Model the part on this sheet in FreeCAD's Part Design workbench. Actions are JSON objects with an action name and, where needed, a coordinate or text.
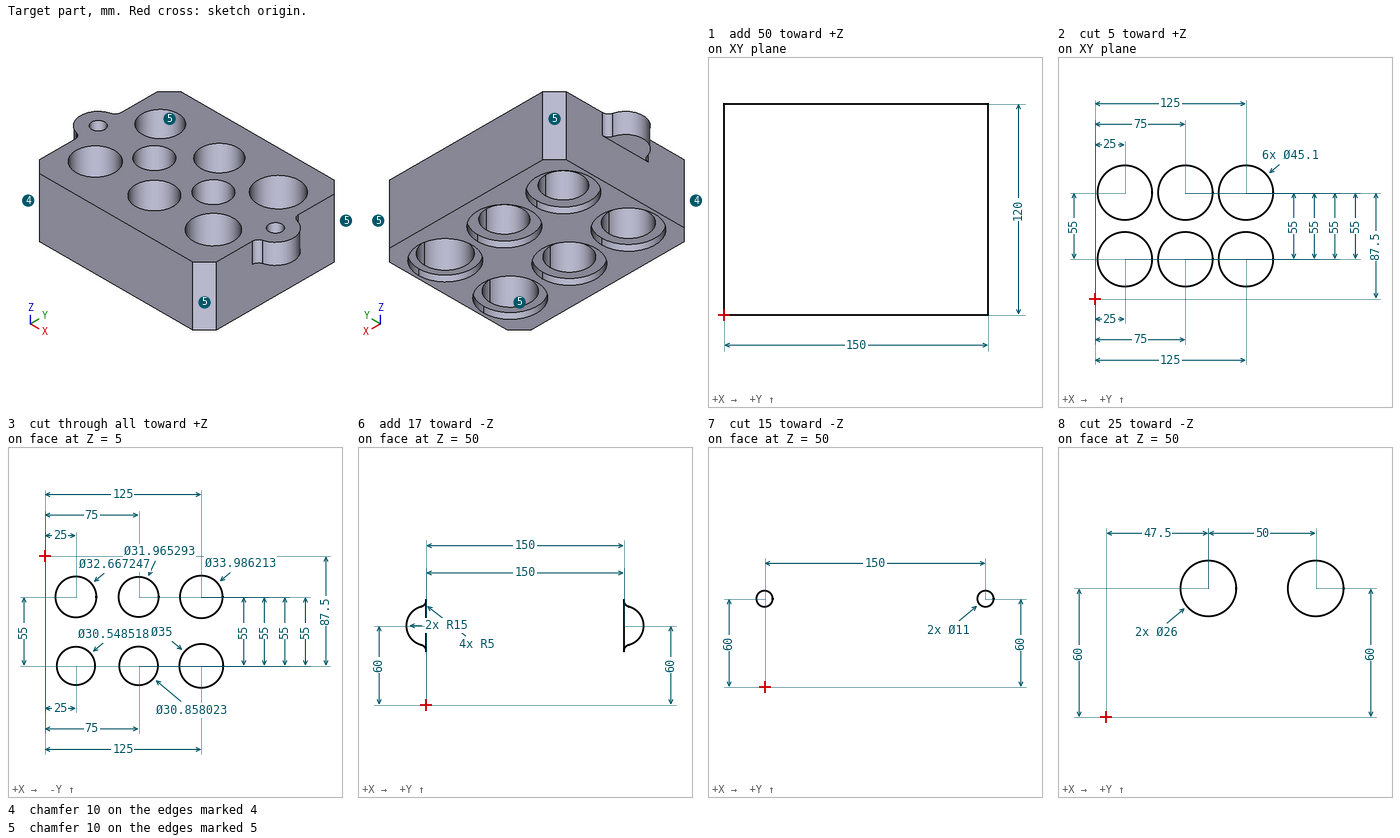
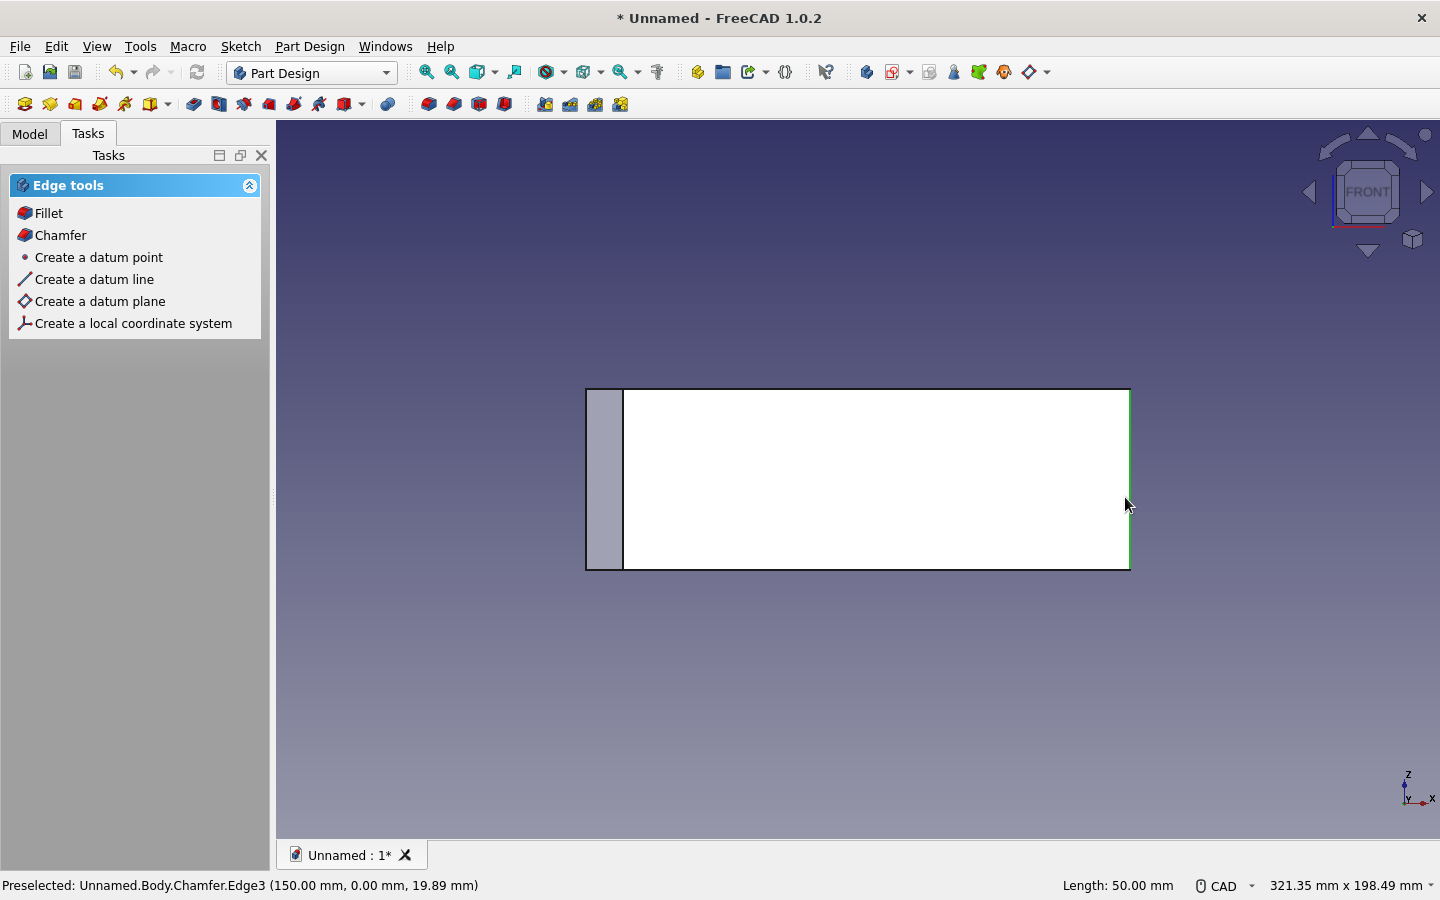
{"action": "key", "text": "3"}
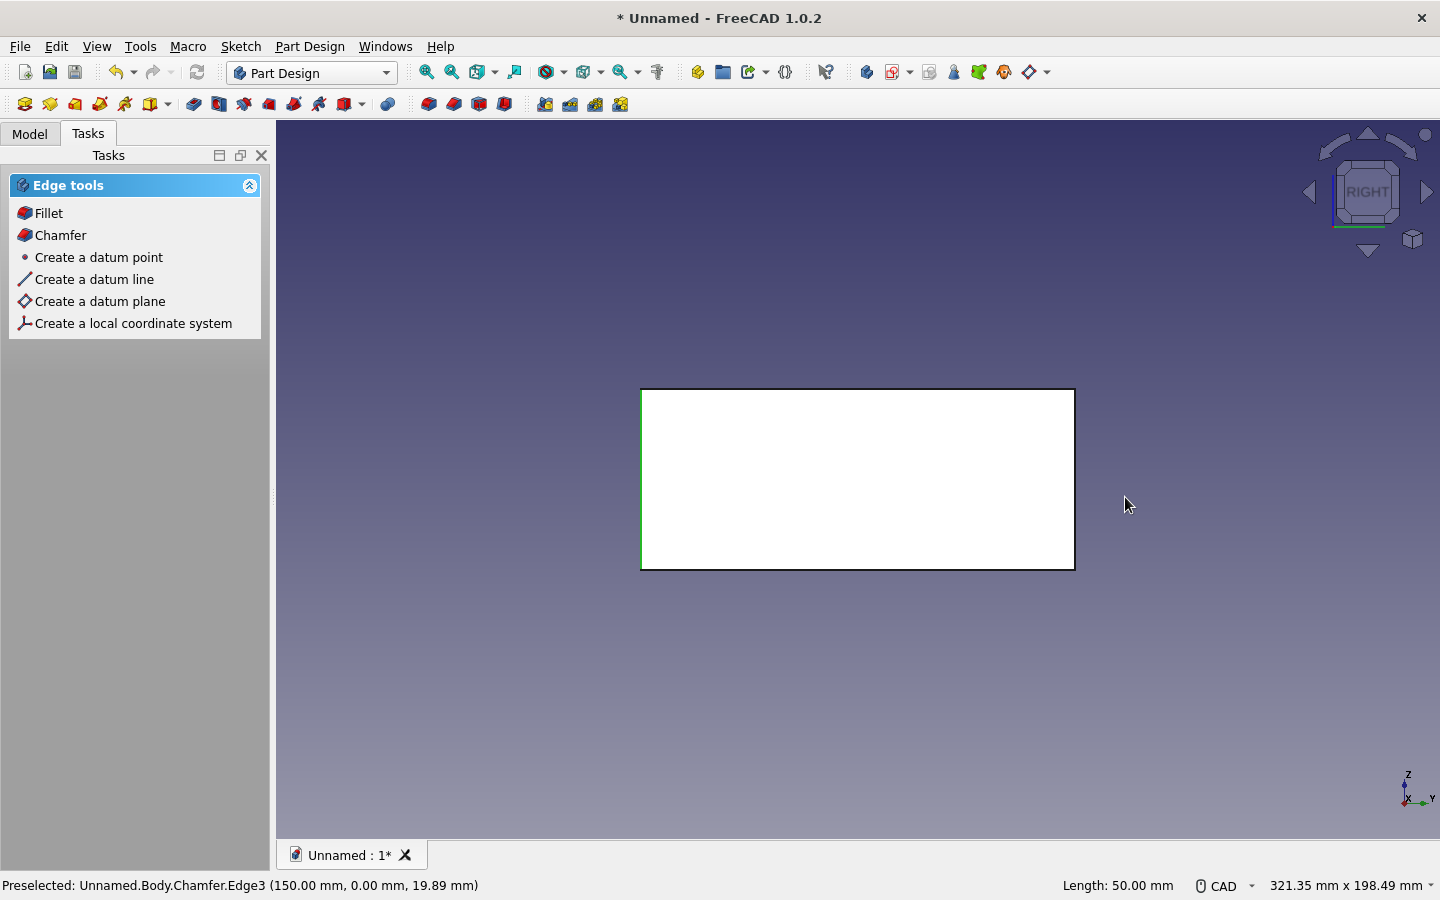
{"action": "left_click", "coordinate": [427, 72]}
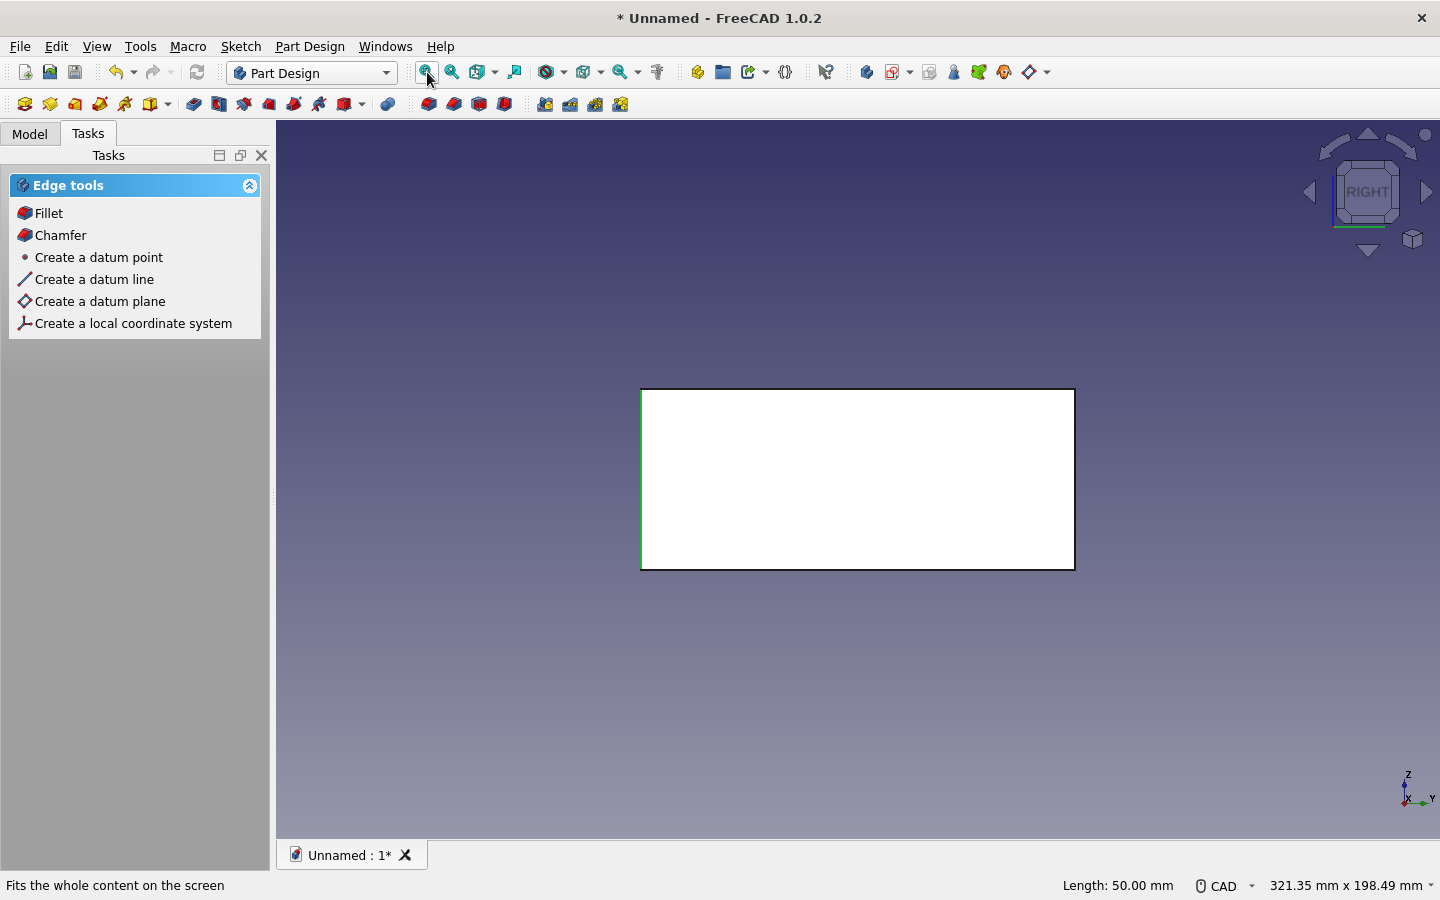
{"action": "left_click", "coordinate": [1075, 478], "text": "ctrl"}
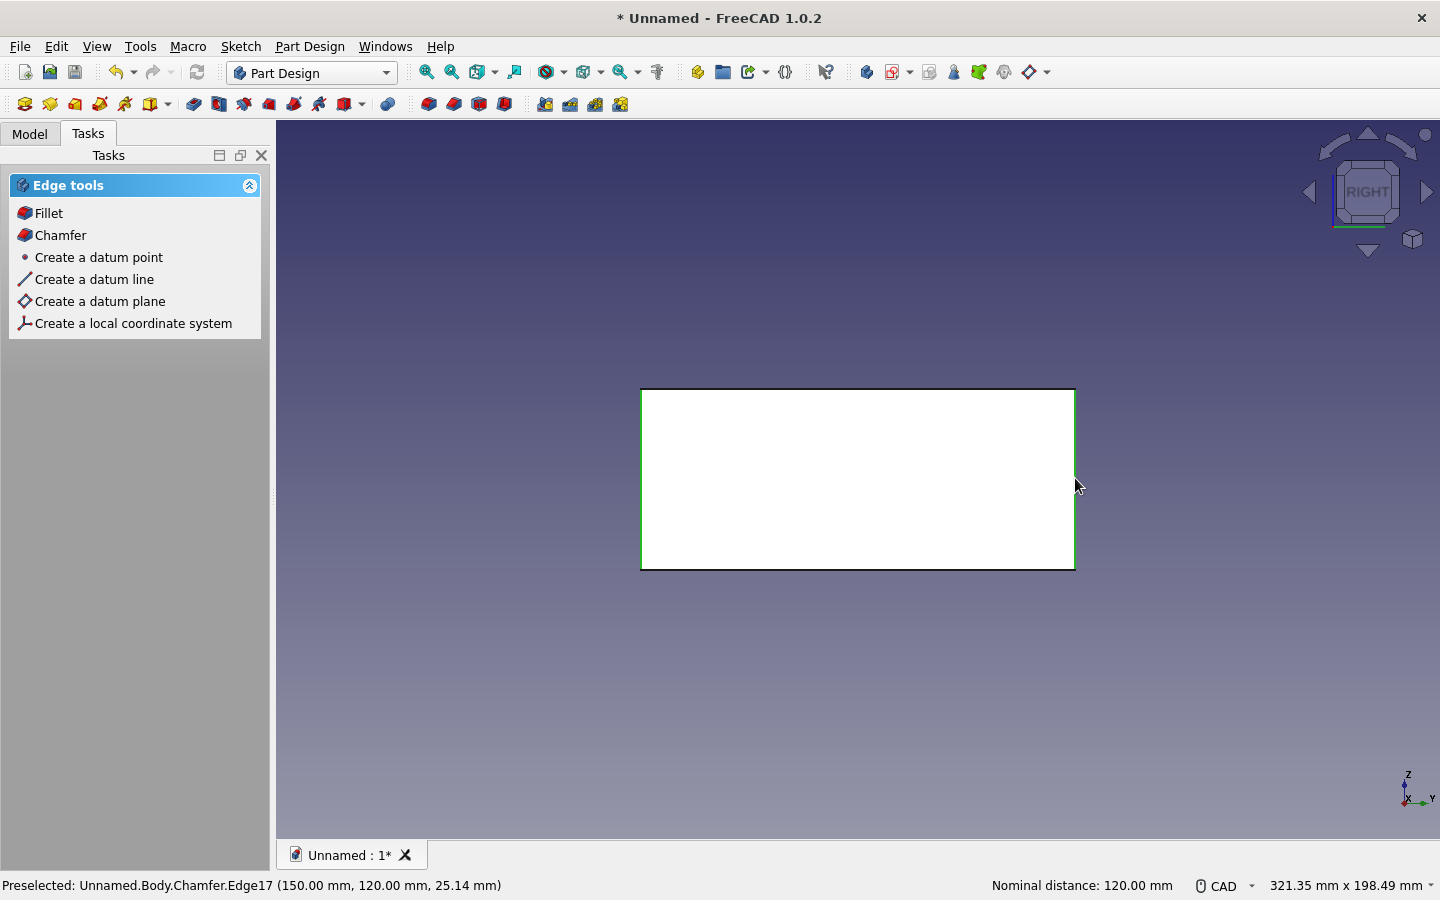
{"action": "key", "text": "5"}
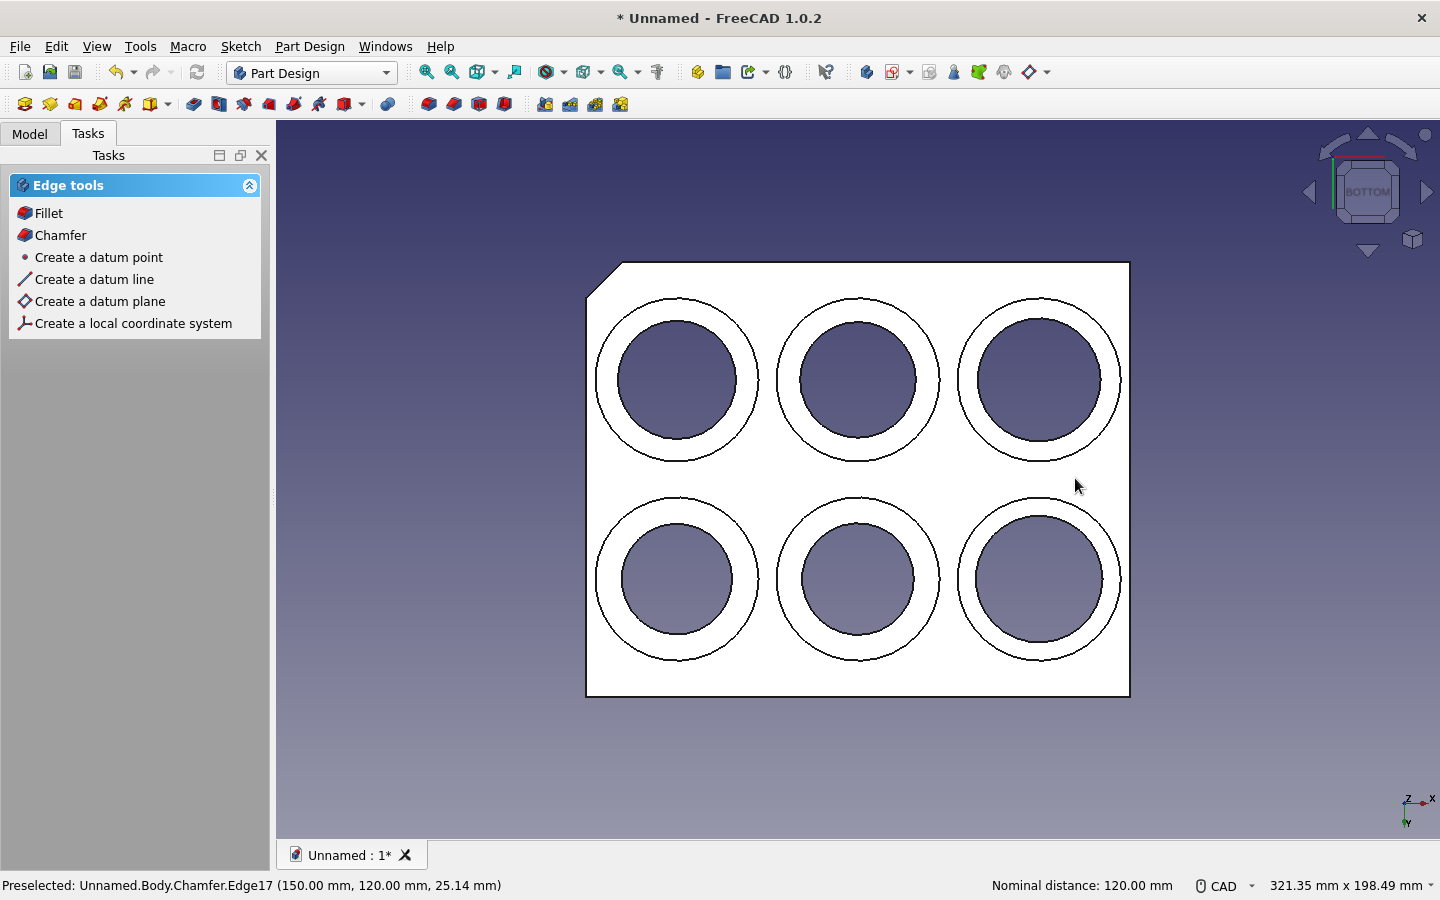
{"action": "key", "text": "4"}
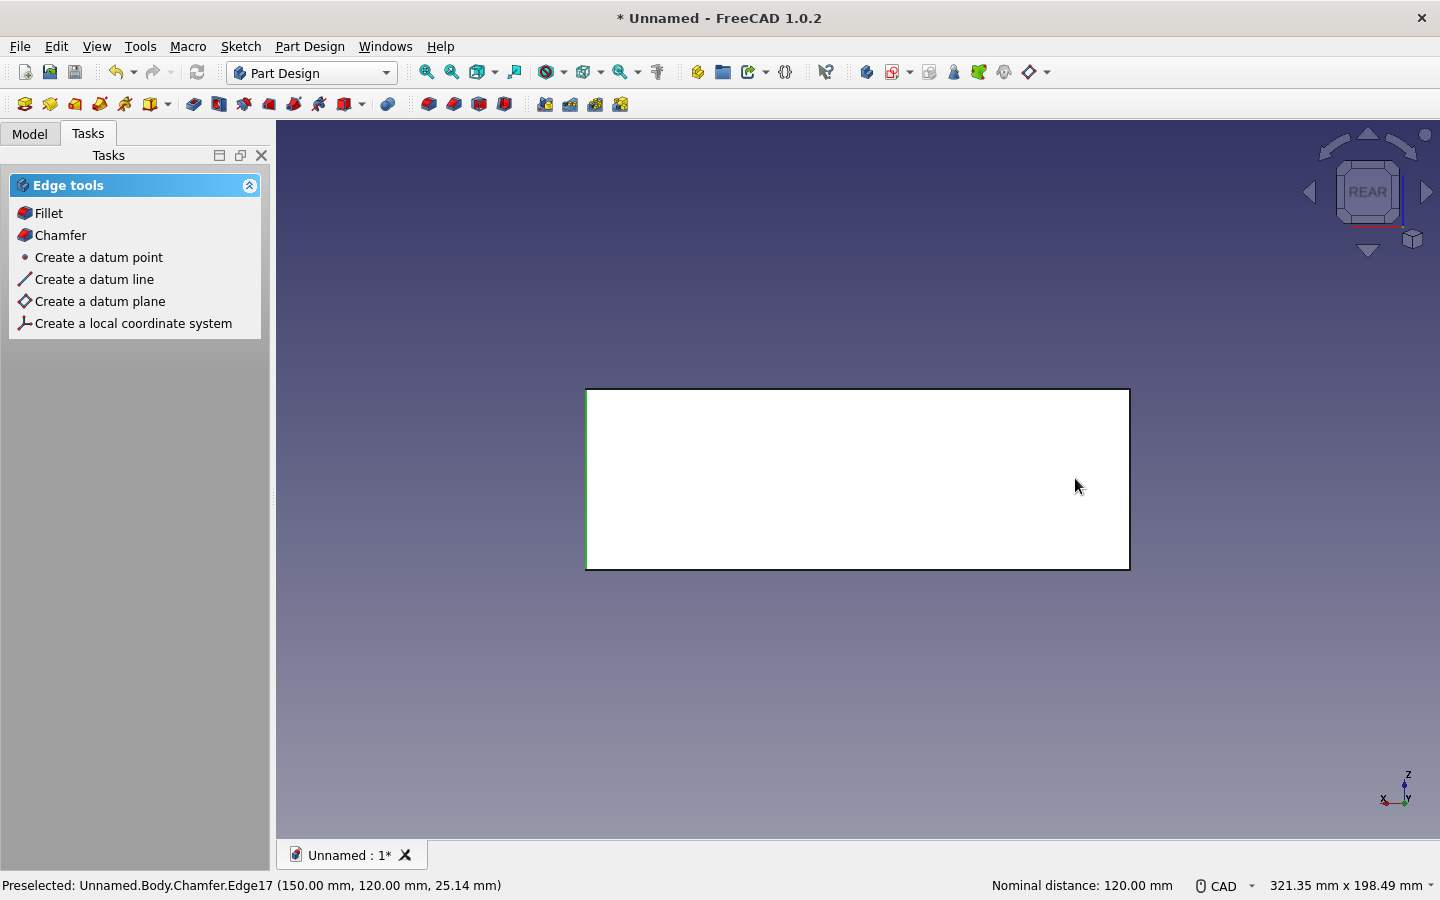
{"action": "left_click", "coordinate": [1130, 479], "text": "ctrl"}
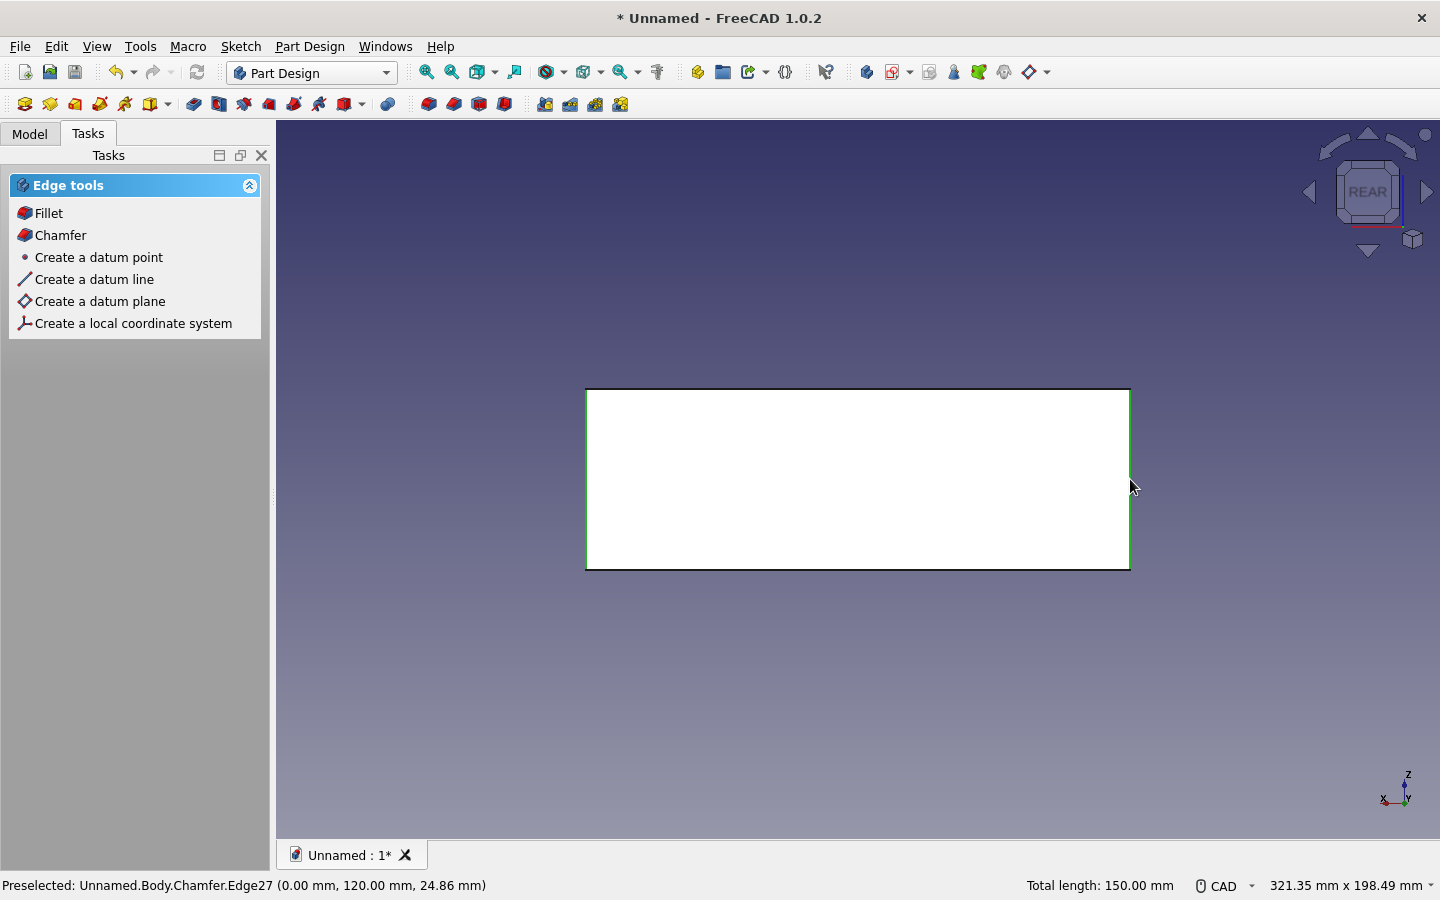
{"action": "left_click", "coordinate": [454, 104]}